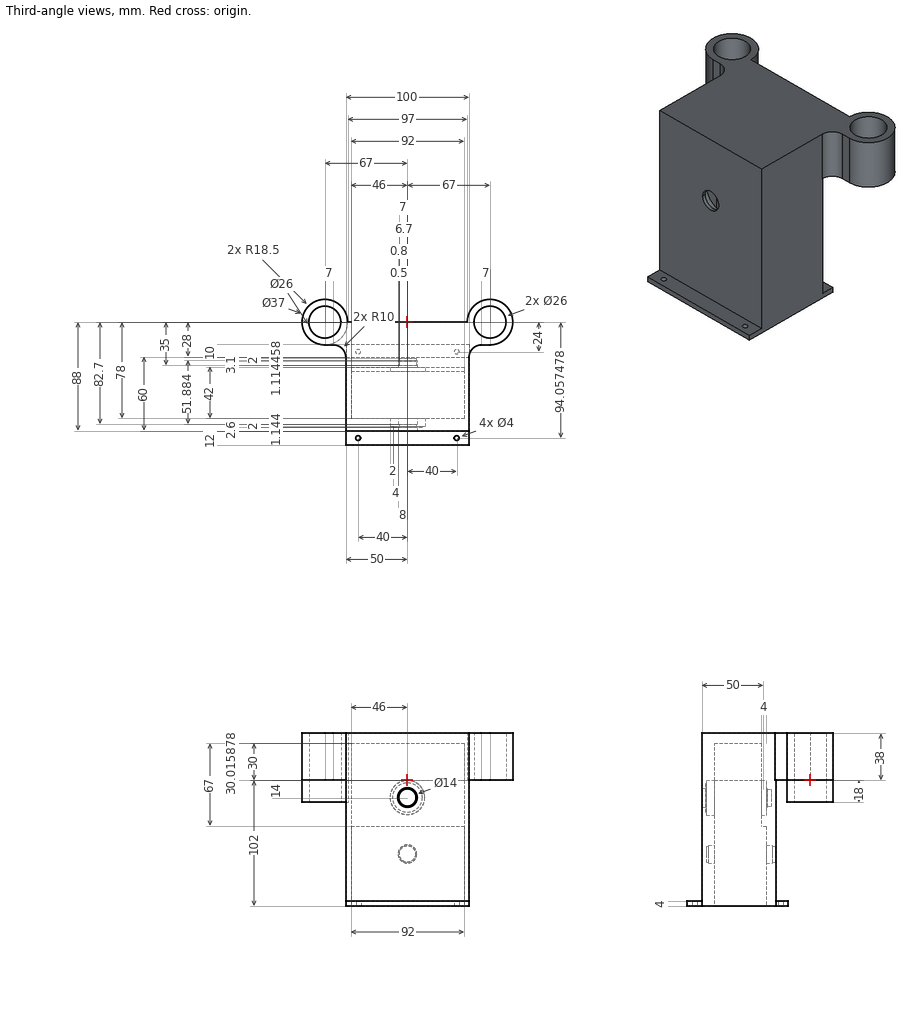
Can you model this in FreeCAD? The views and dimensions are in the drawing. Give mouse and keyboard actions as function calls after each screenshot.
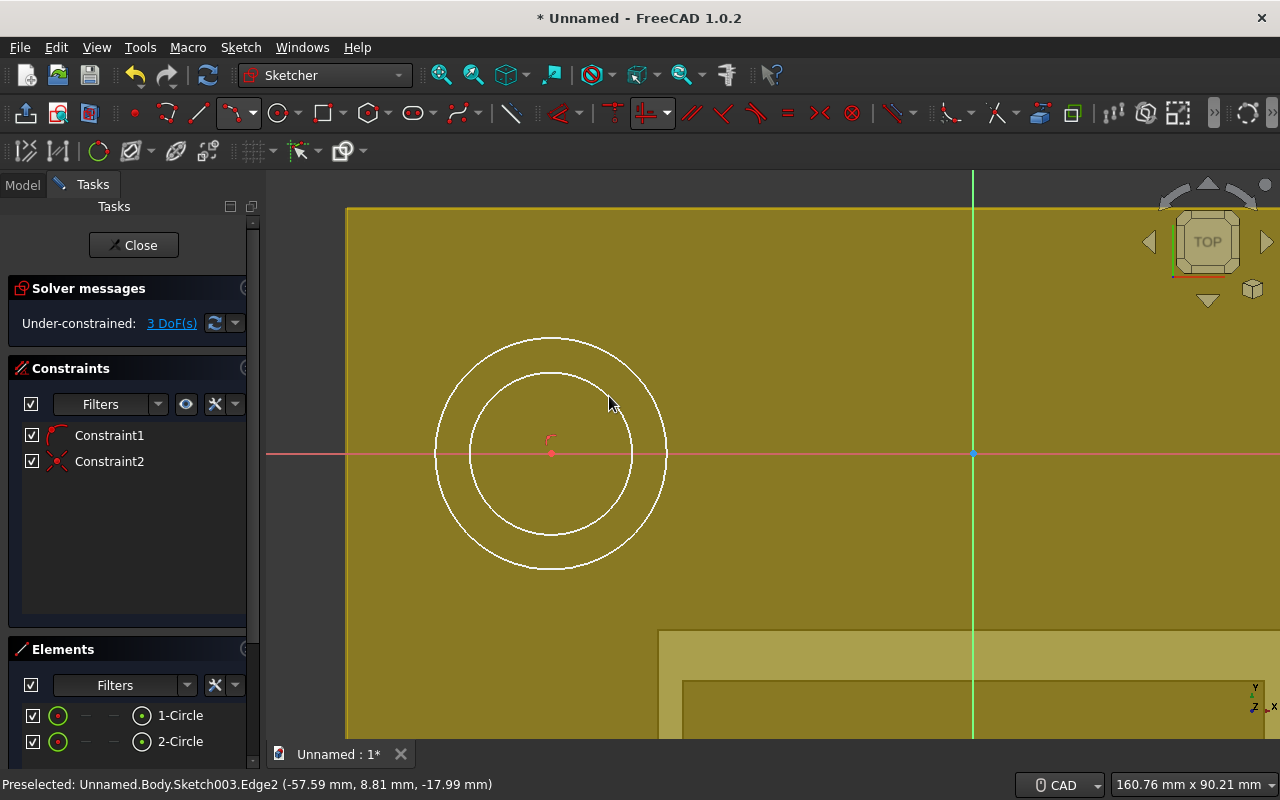
click(558, 114)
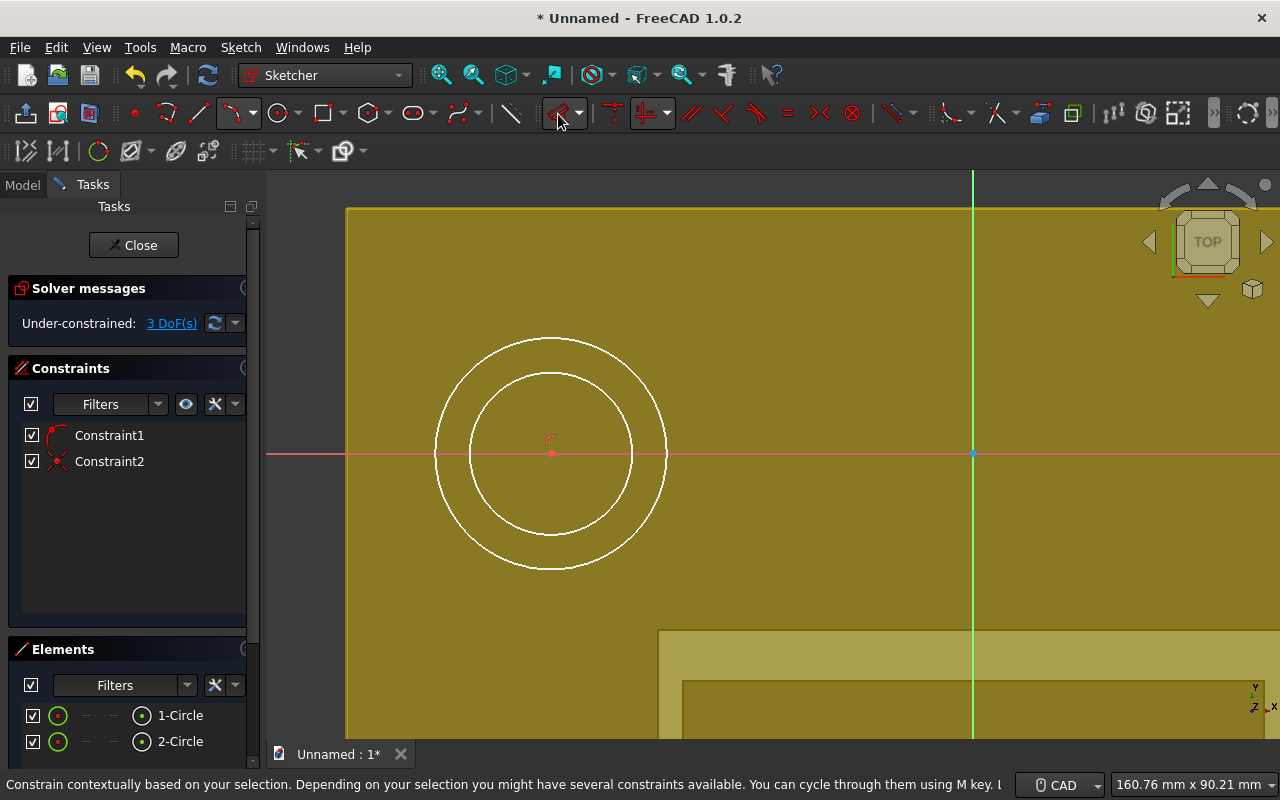
click(633, 372)
click(656, 349)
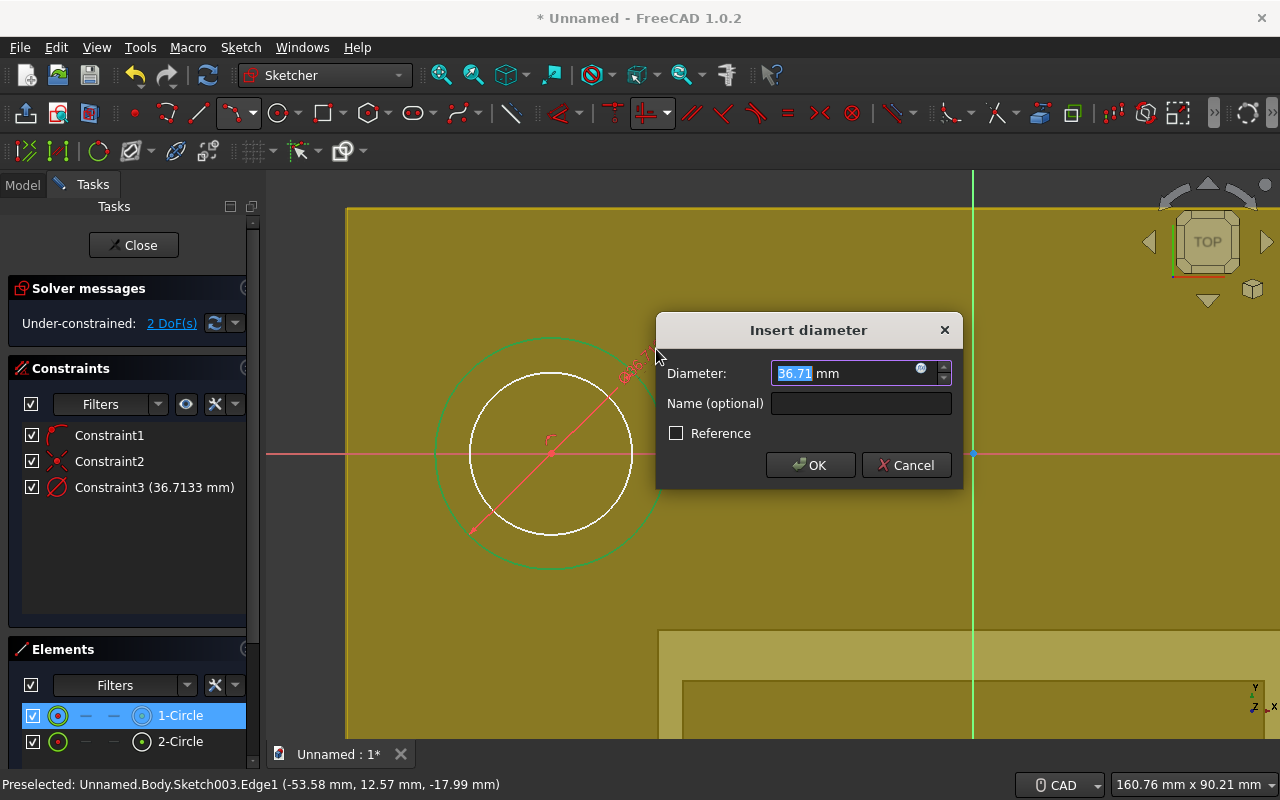
text(37)
key(Return)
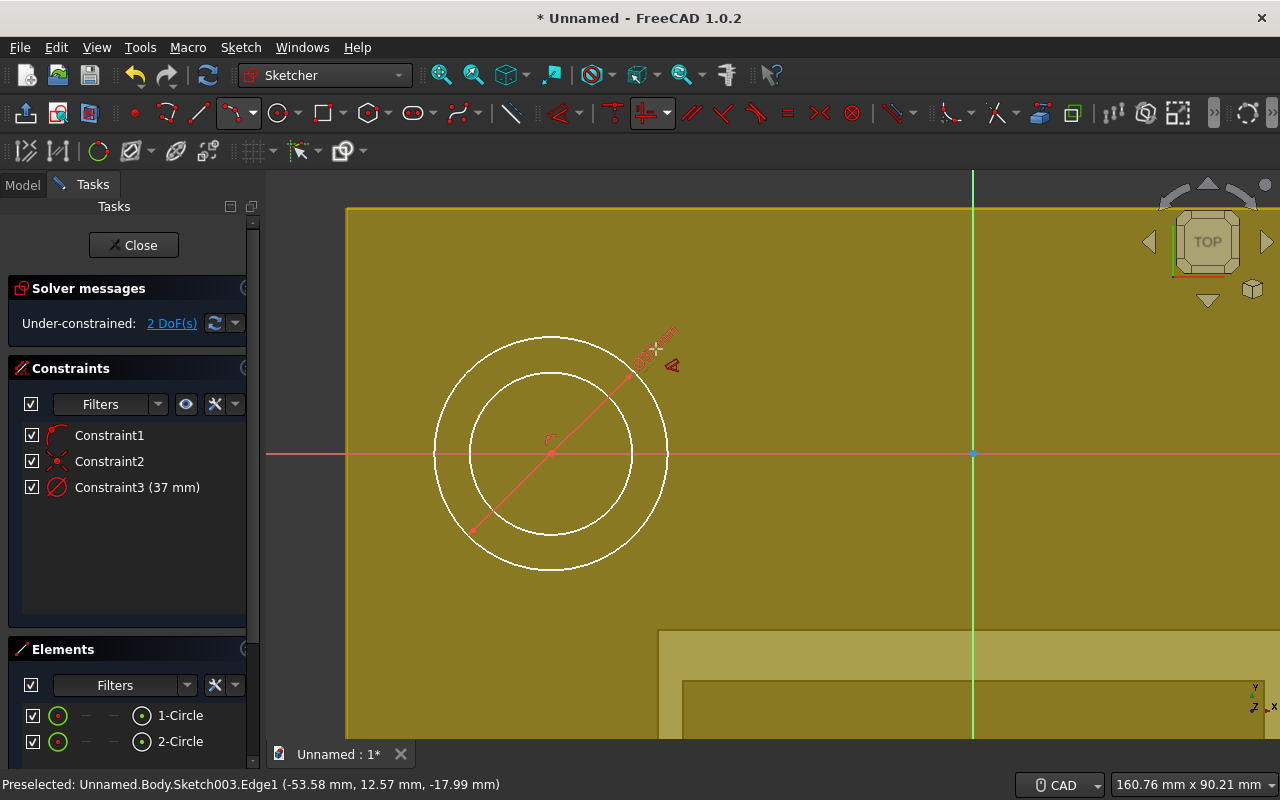
click(608, 396)
click(681, 415)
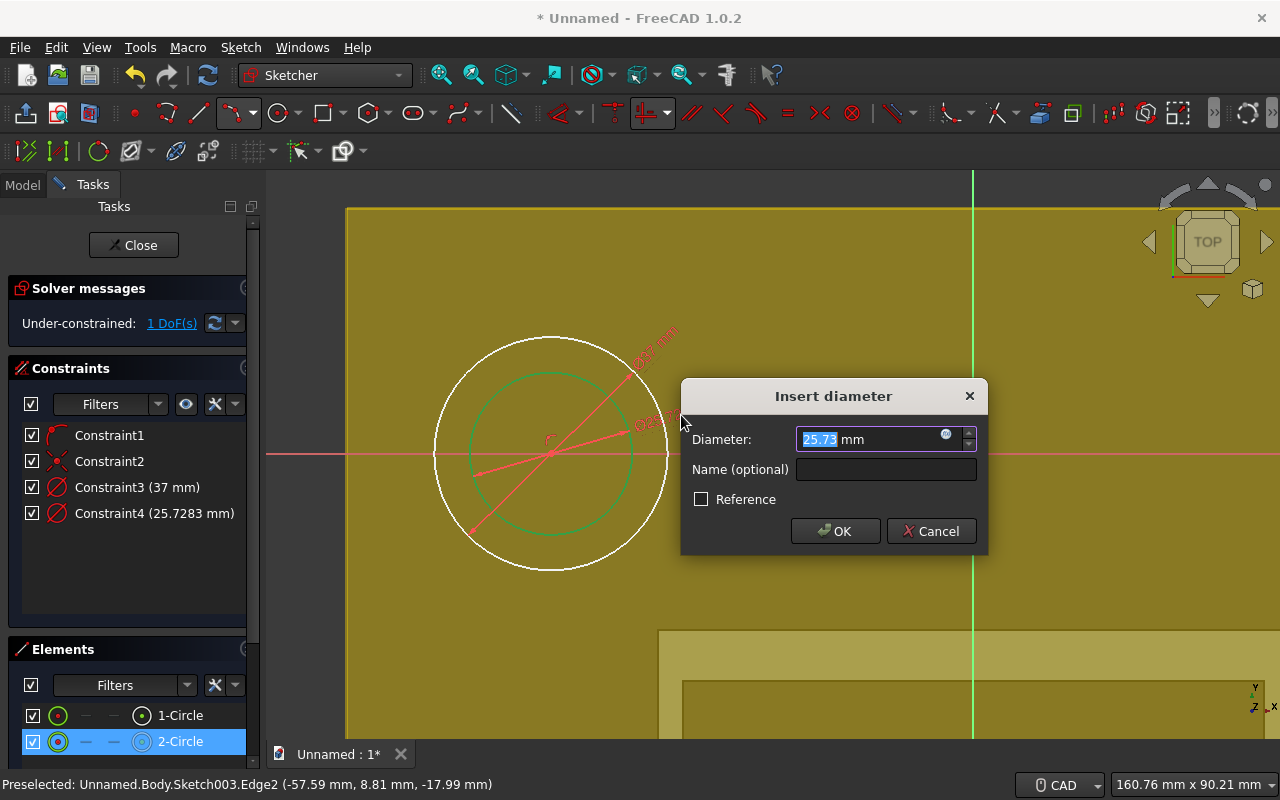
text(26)
key(Return)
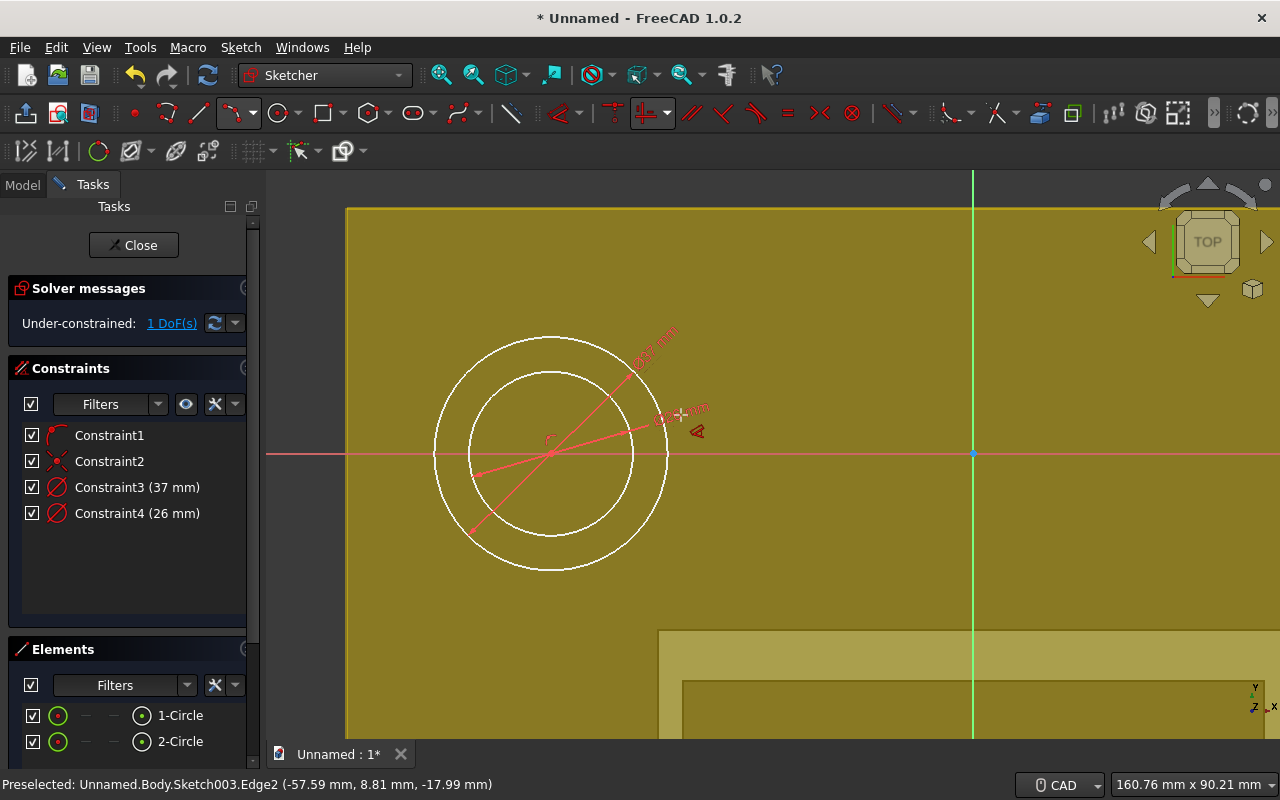
click(551, 454)
click(762, 488)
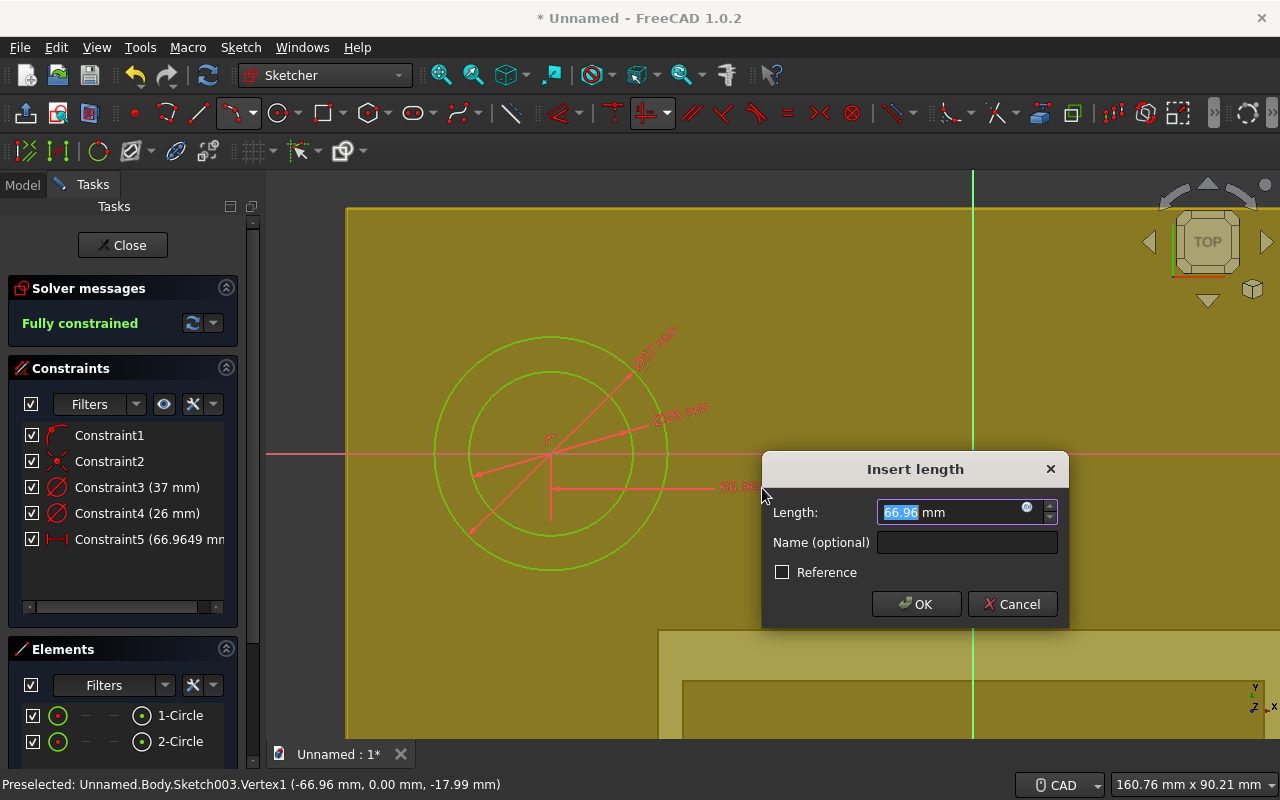
text(67)
key(Return)
key(Escape)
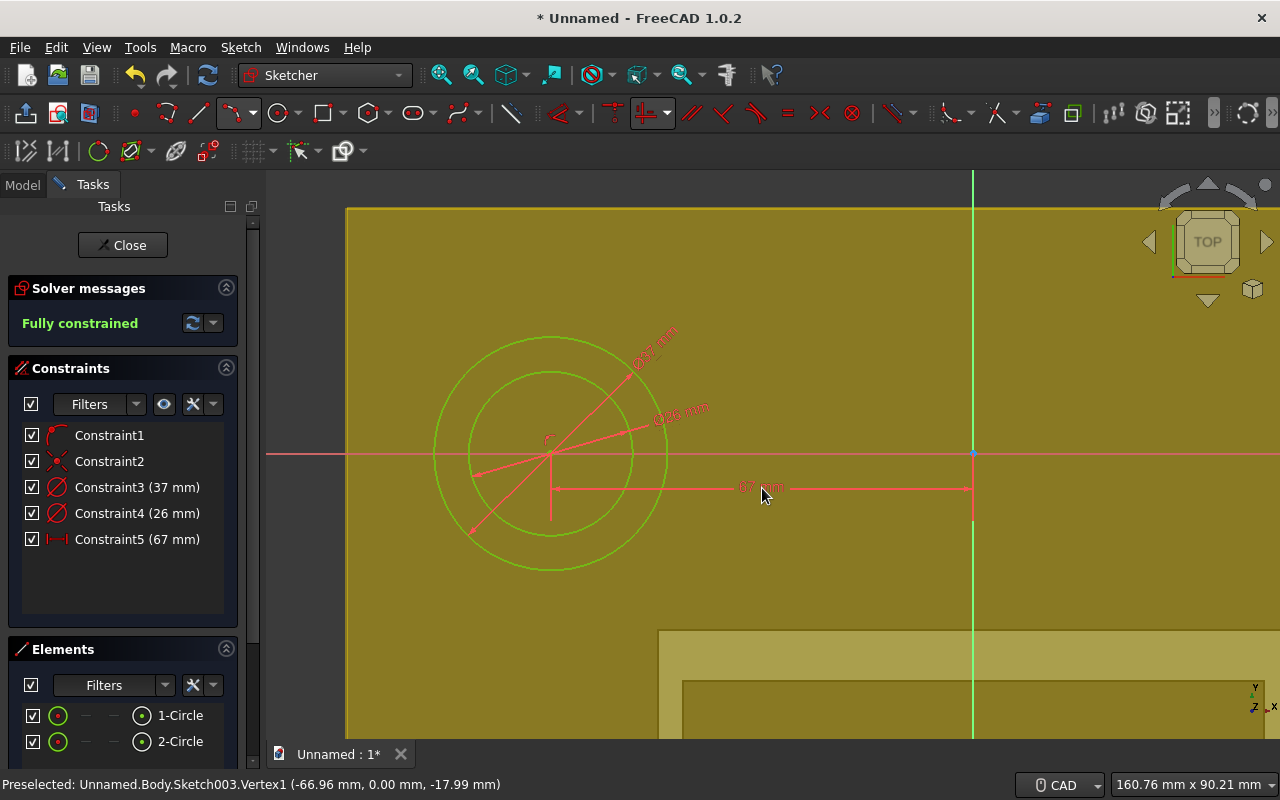
click(123, 245)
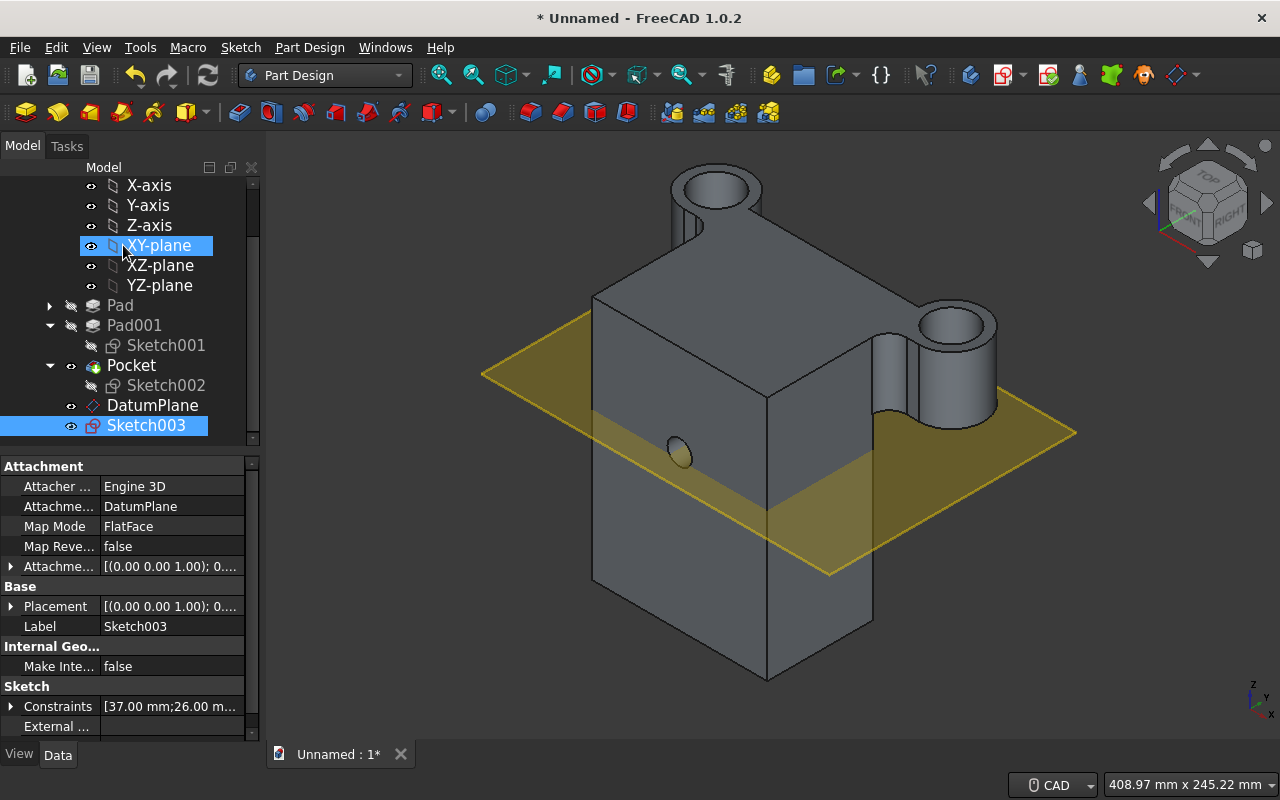
click(26, 112)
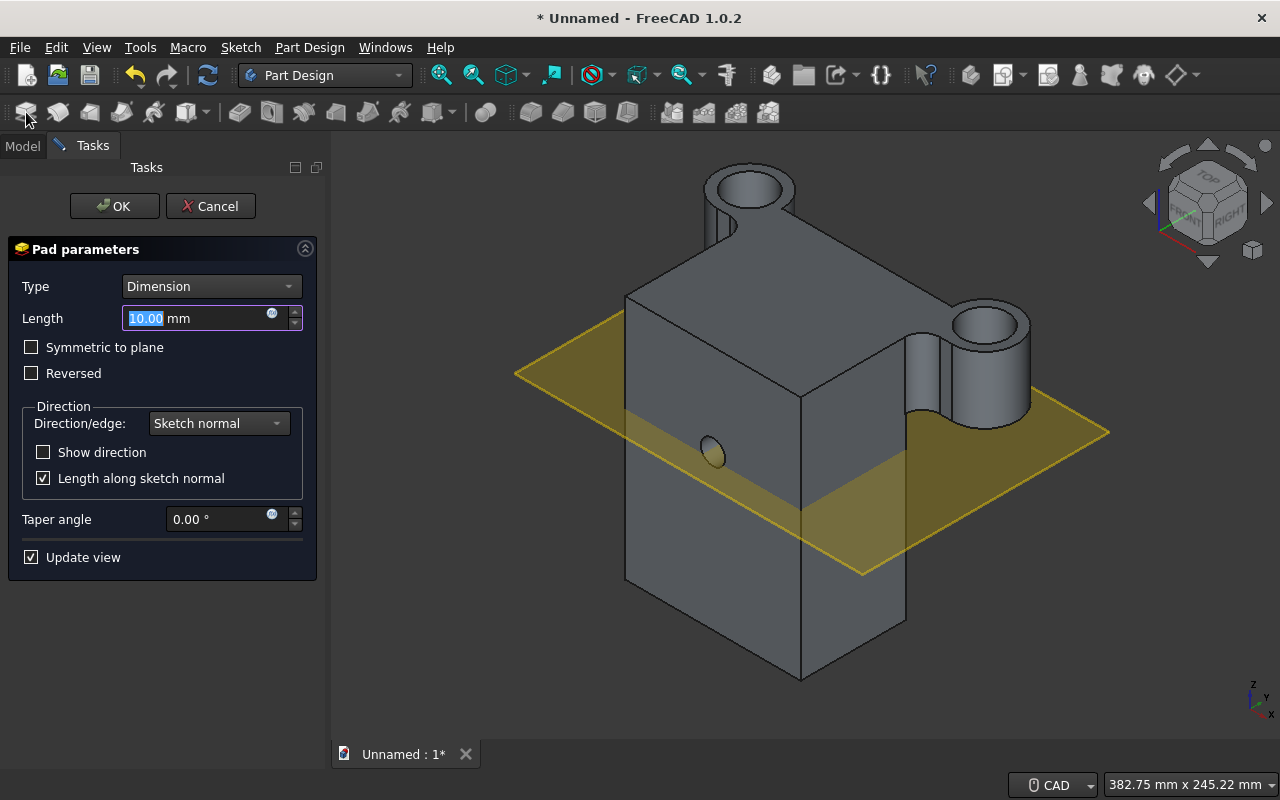
text(18)
key(Tab)